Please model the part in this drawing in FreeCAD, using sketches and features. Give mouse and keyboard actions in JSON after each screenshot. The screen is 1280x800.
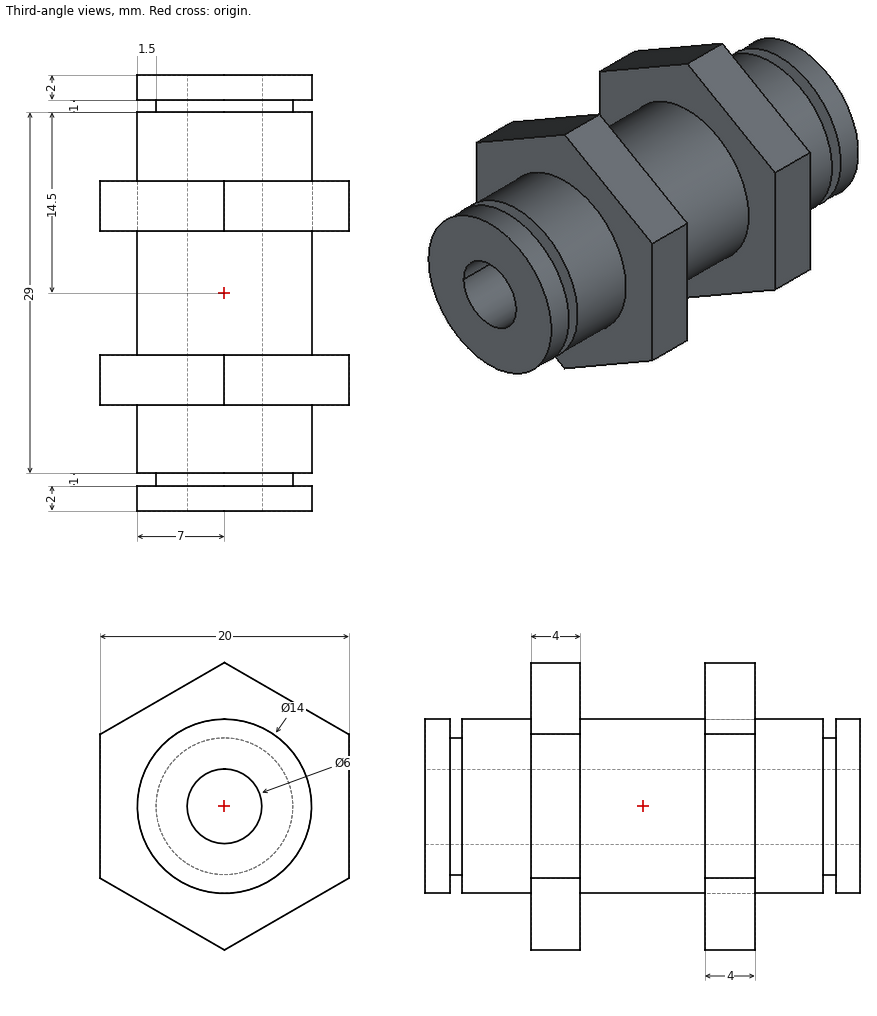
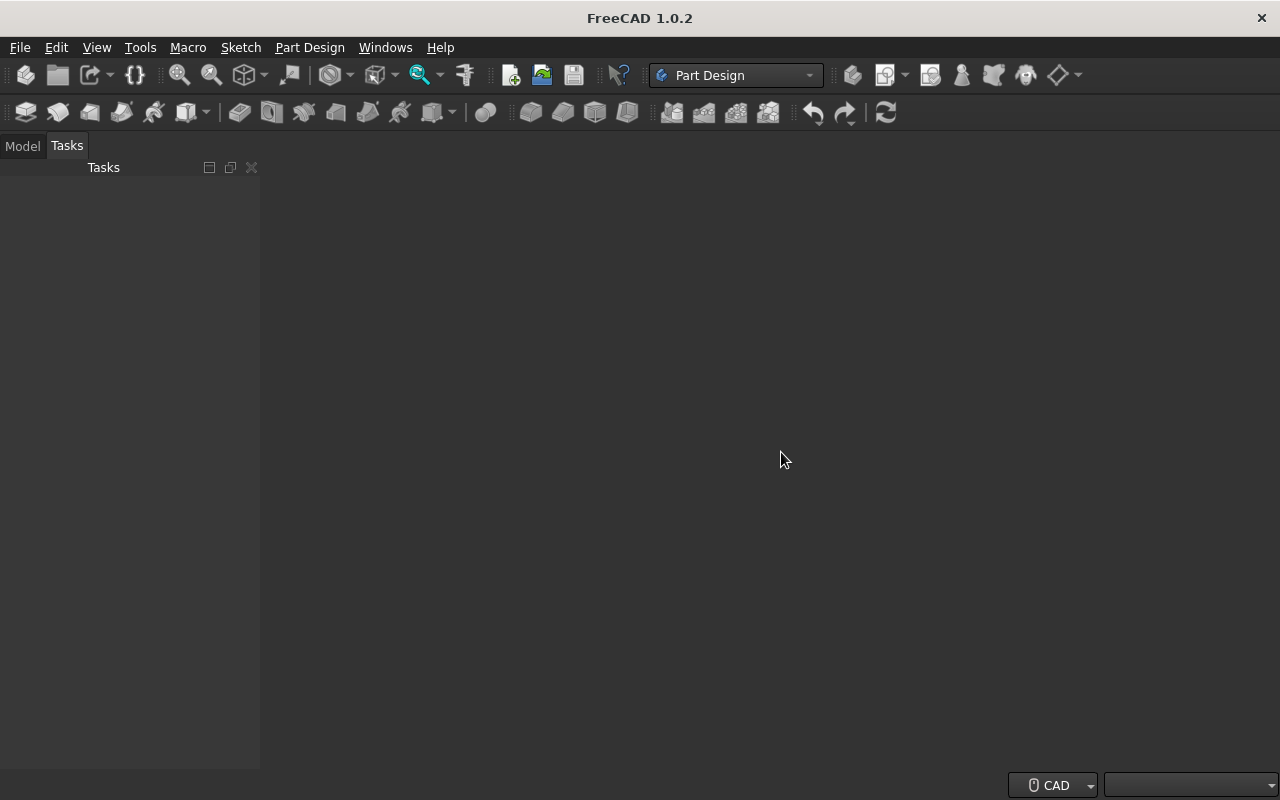
{"action": "left_click", "coordinate": [510, 76]}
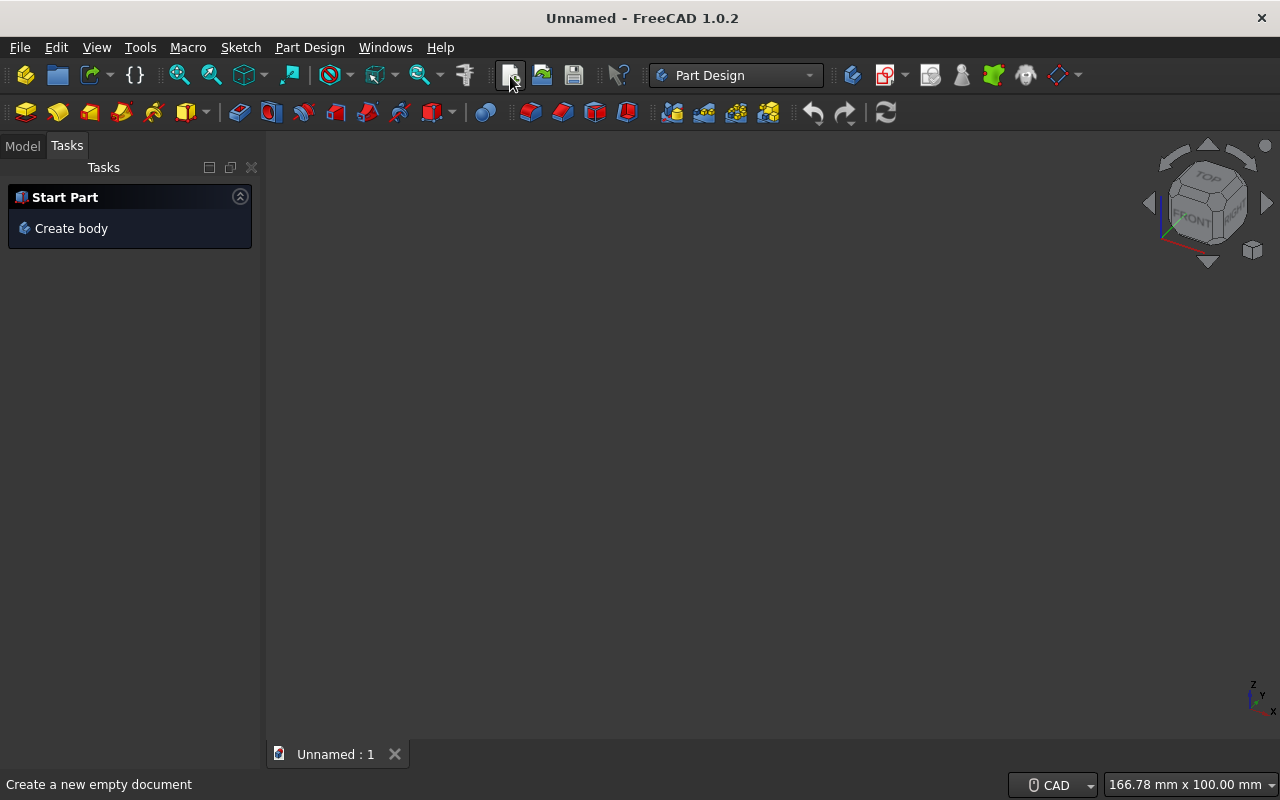
{"action": "left_click", "coordinate": [886, 76]}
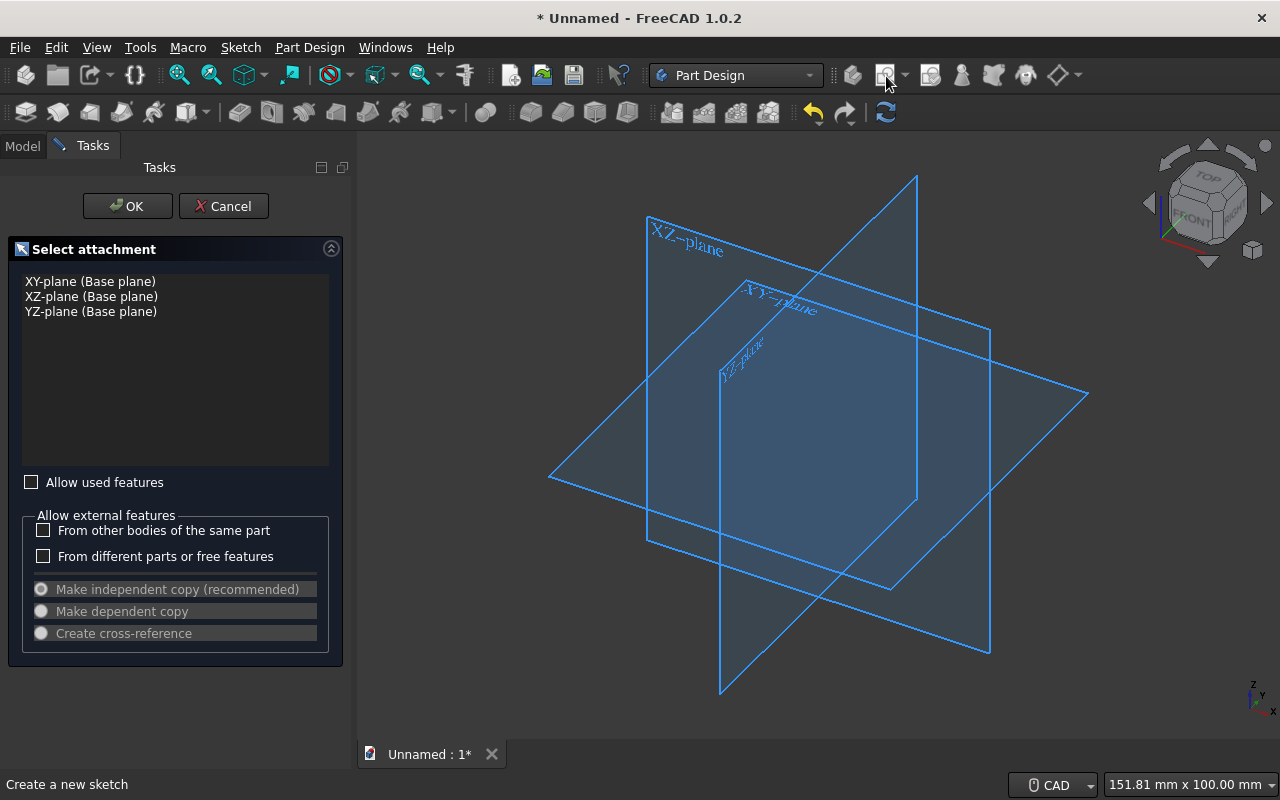
{"action": "left_click", "coordinate": [82, 282]}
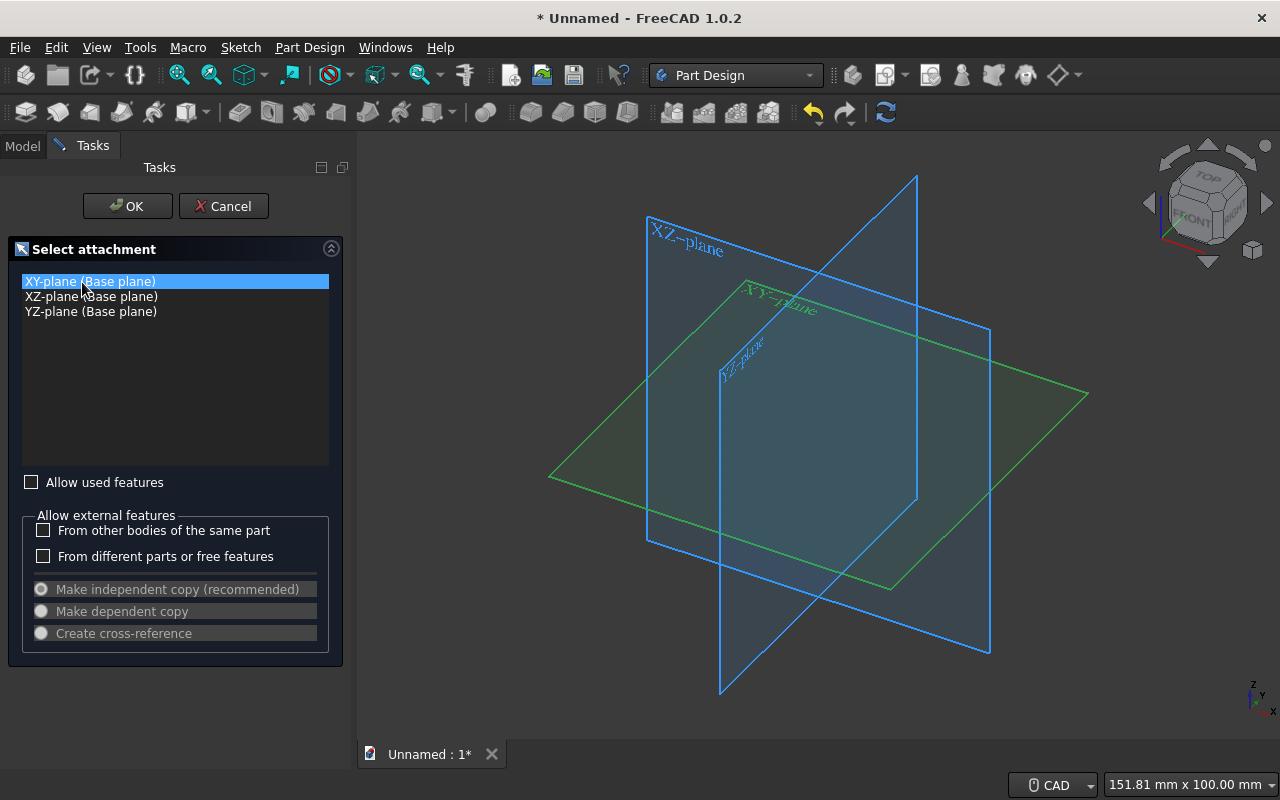
{"action": "left_click", "coordinate": [128, 206]}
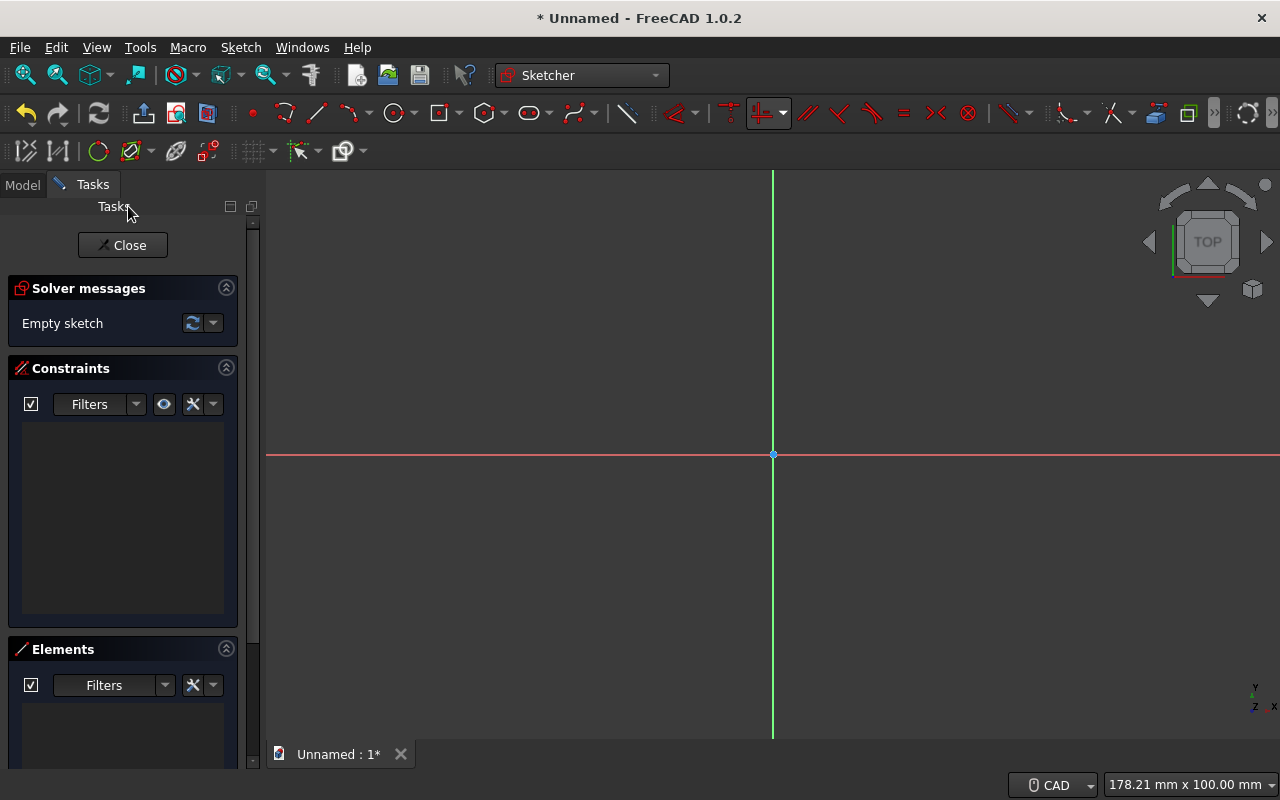
{"action": "scroll", "coordinate": [812, 454], "scroll_direction": "up", "scroll_amount": 3}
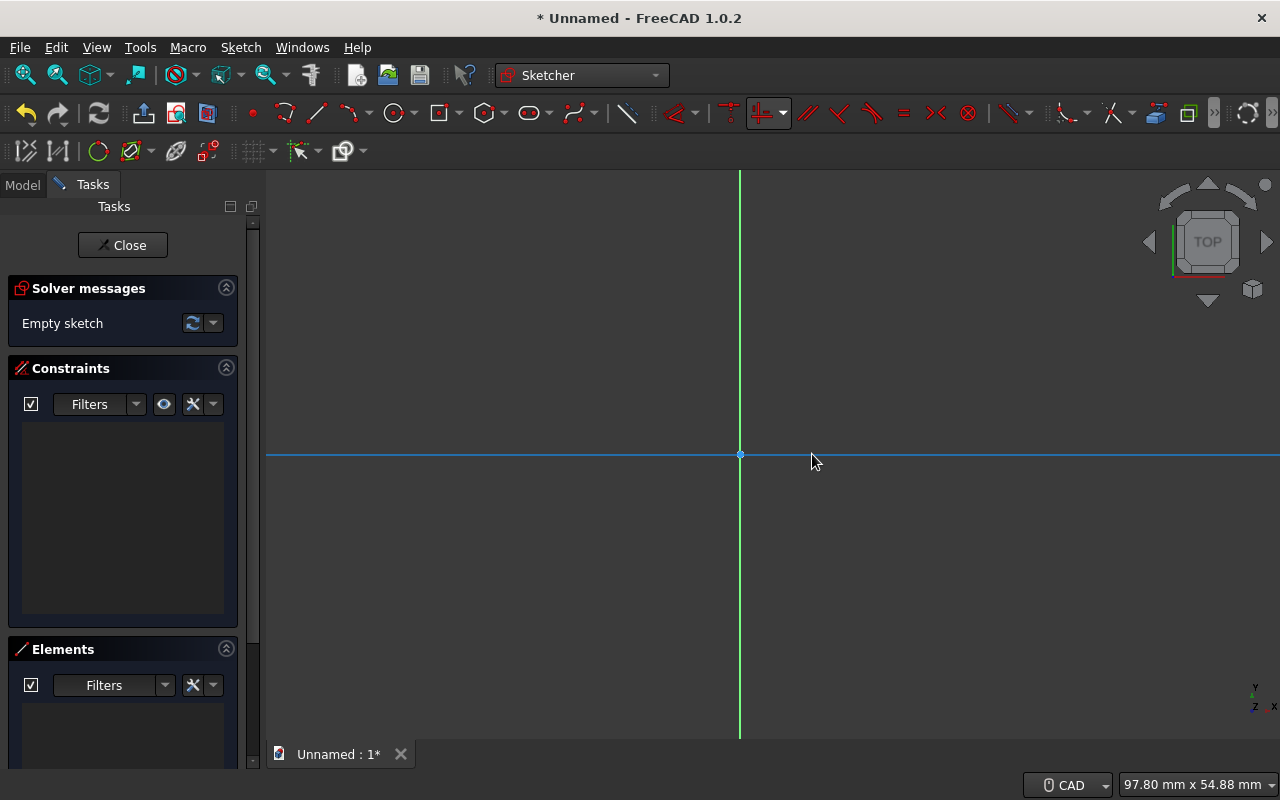
{"action": "left_click", "coordinate": [286, 114]}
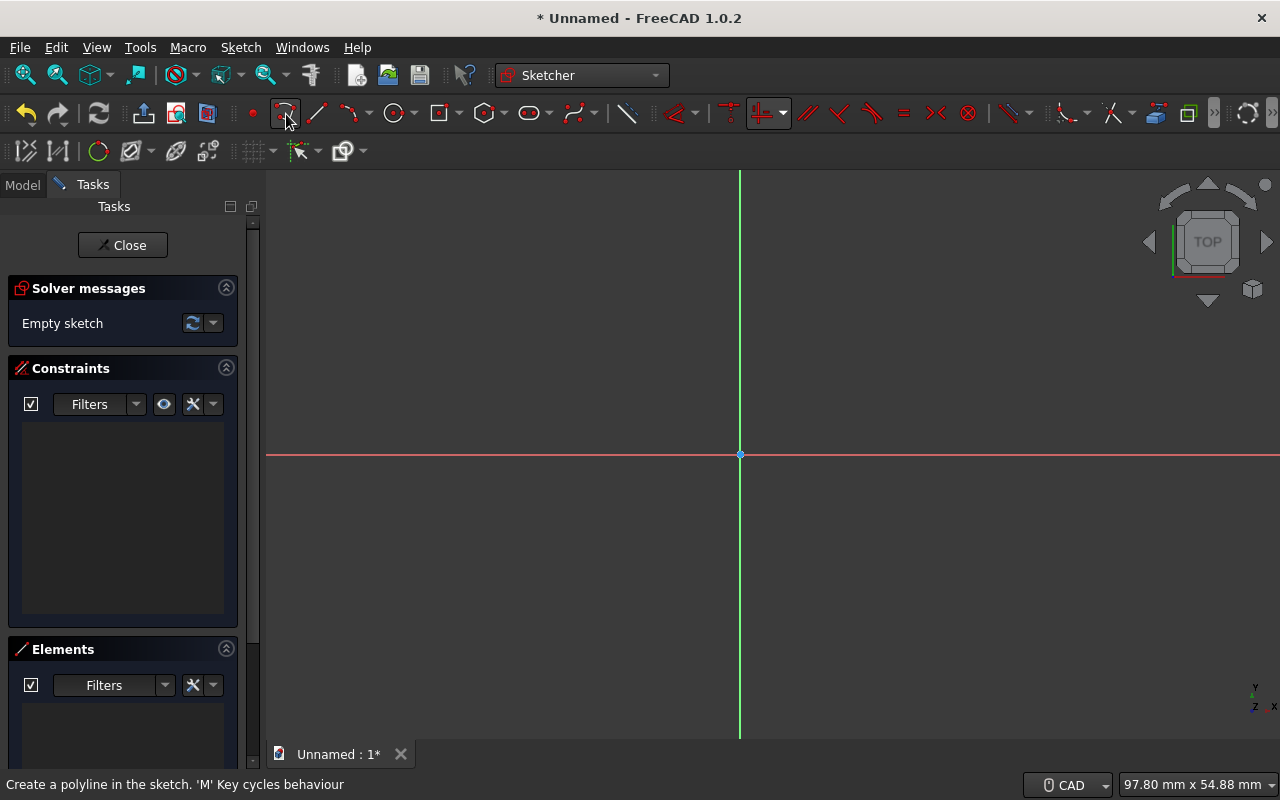
{"action": "left_click", "coordinate": [683, 304]}
{"action": "left_click", "coordinate": [668, 304]}
{"action": "left_click", "coordinate": [668, 605]}
{"action": "left_click", "coordinate": [683, 605]}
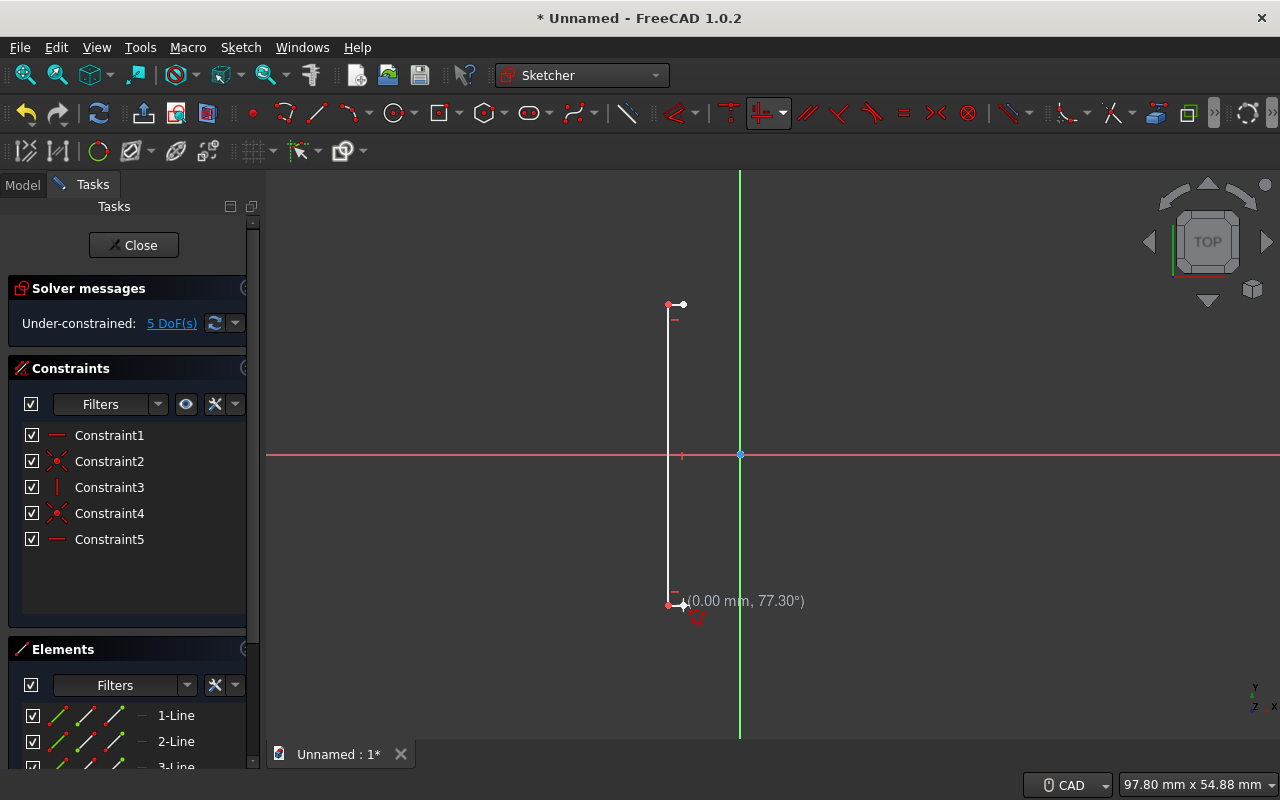
{"action": "scroll", "coordinate": [683, 615], "scroll_direction": "up", "scroll_amount": 3}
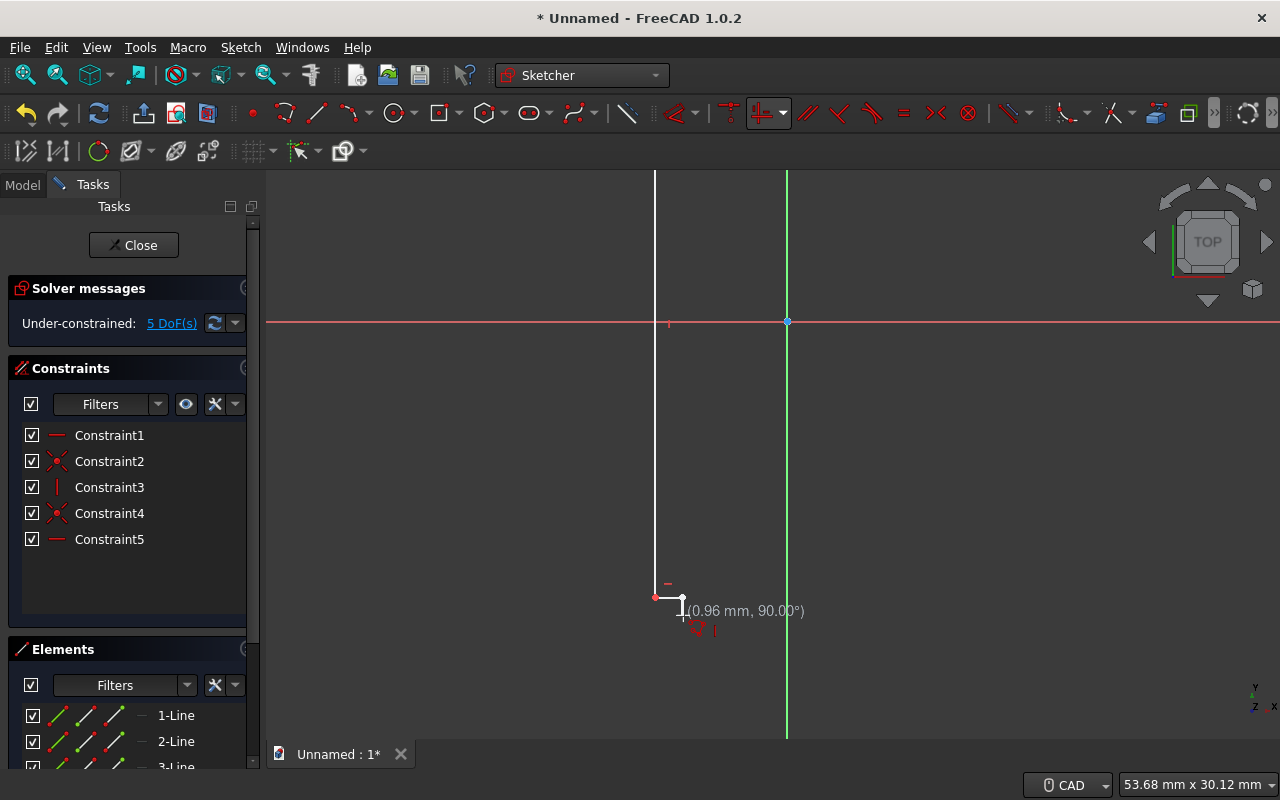
{"action": "left_click", "coordinate": [683, 615]}
{"action": "left_click", "coordinate": [655, 615]}
{"action": "left_click", "coordinate": [655, 653]}
{"action": "left_click", "coordinate": [787, 653]}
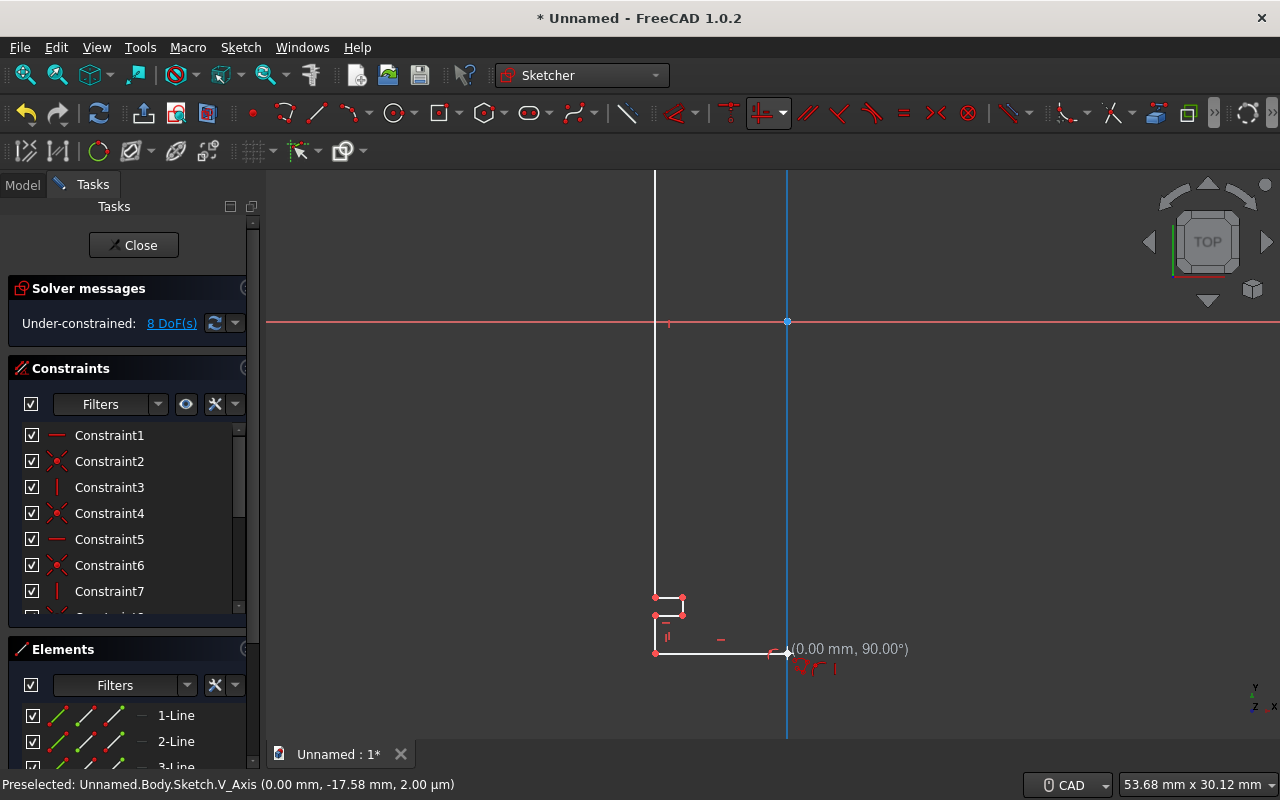
{"action": "scroll", "coordinate": [684, 616], "scroll_direction": "down", "scroll_amount": 3}